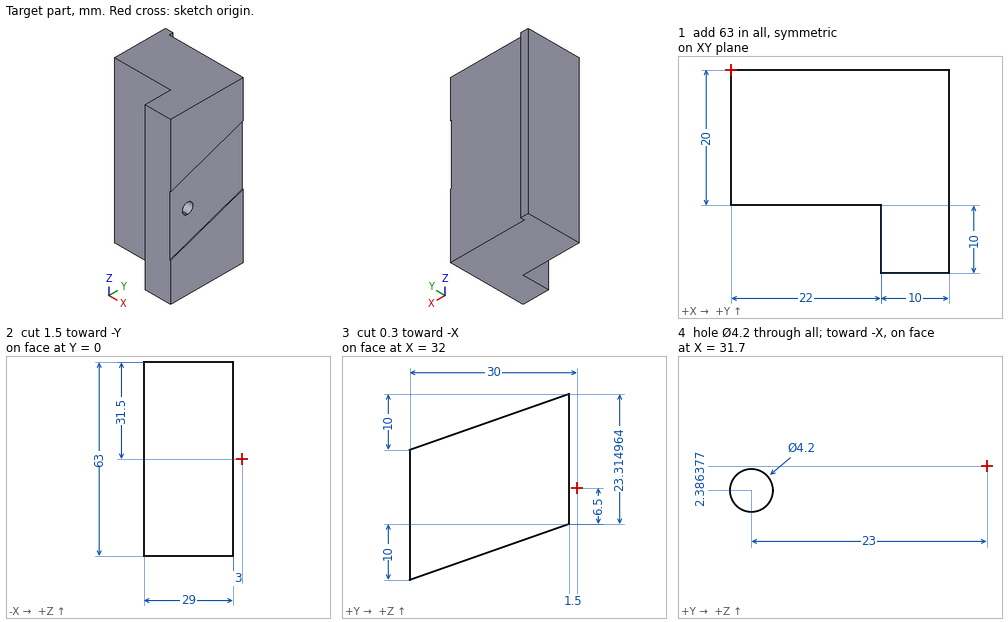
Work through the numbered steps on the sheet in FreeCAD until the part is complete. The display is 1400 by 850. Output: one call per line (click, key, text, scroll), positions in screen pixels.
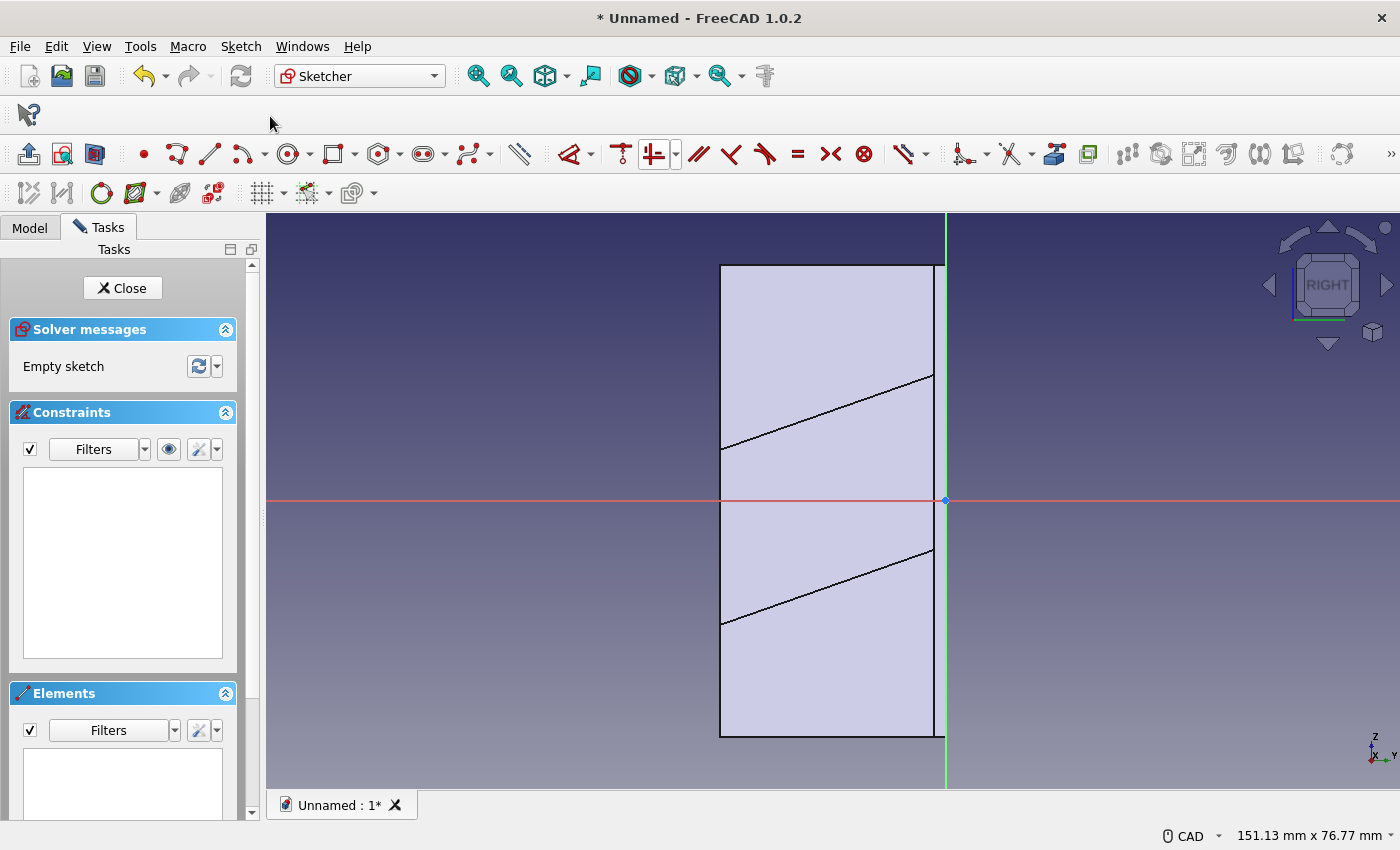
scroll(774, 521, up, 12)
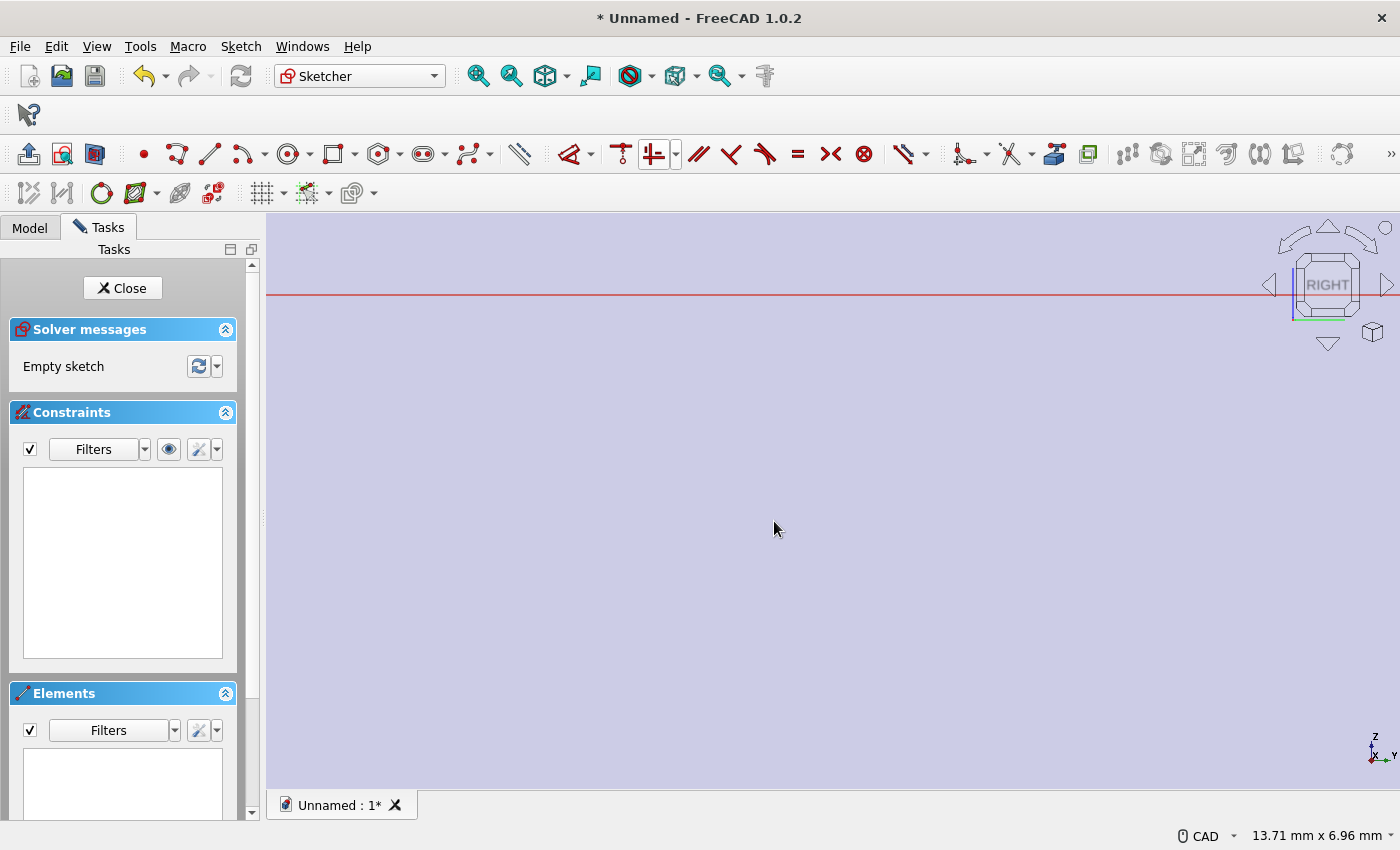
click(288, 154)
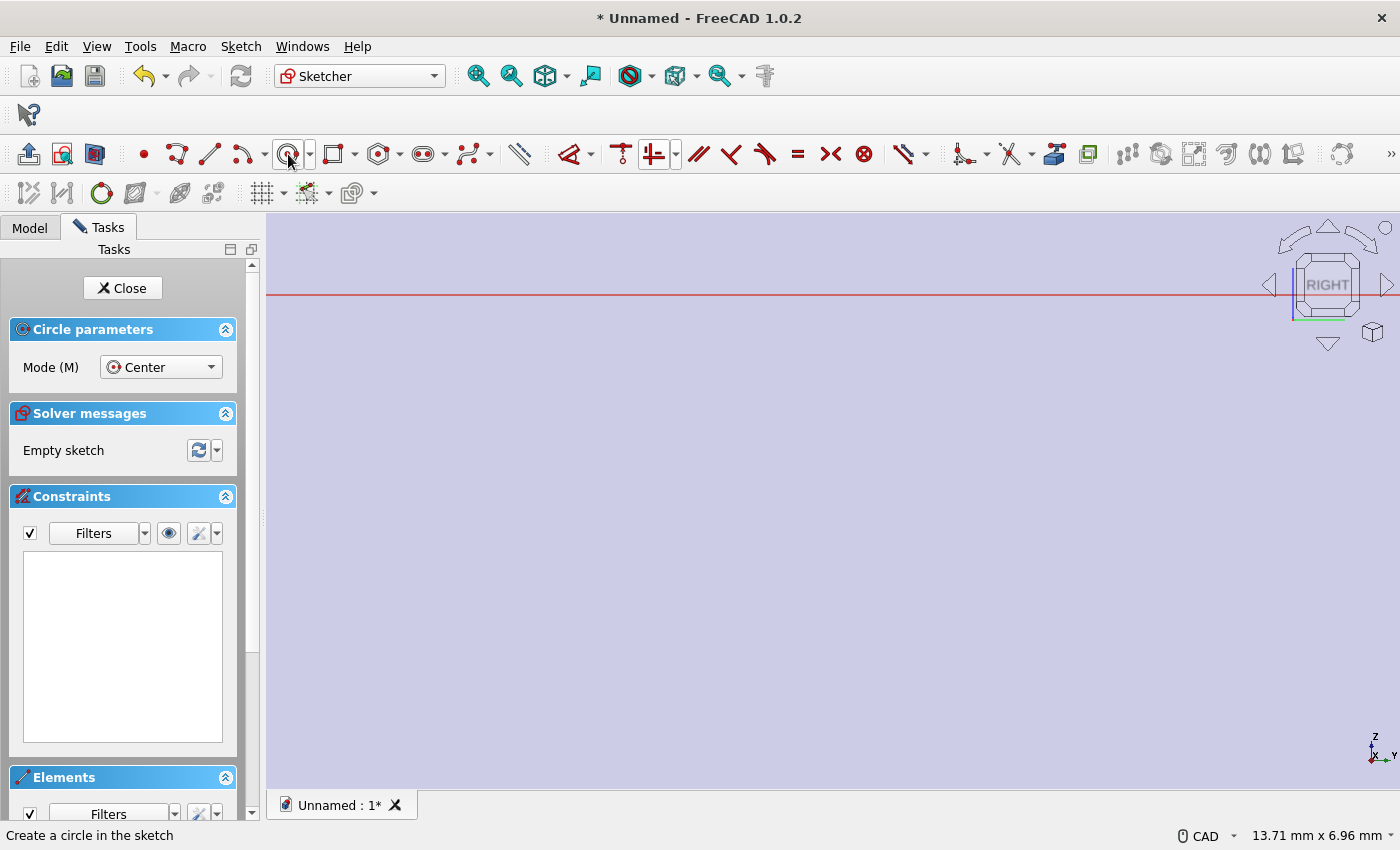
click(758, 493)
click(881, 370)
key(Escape)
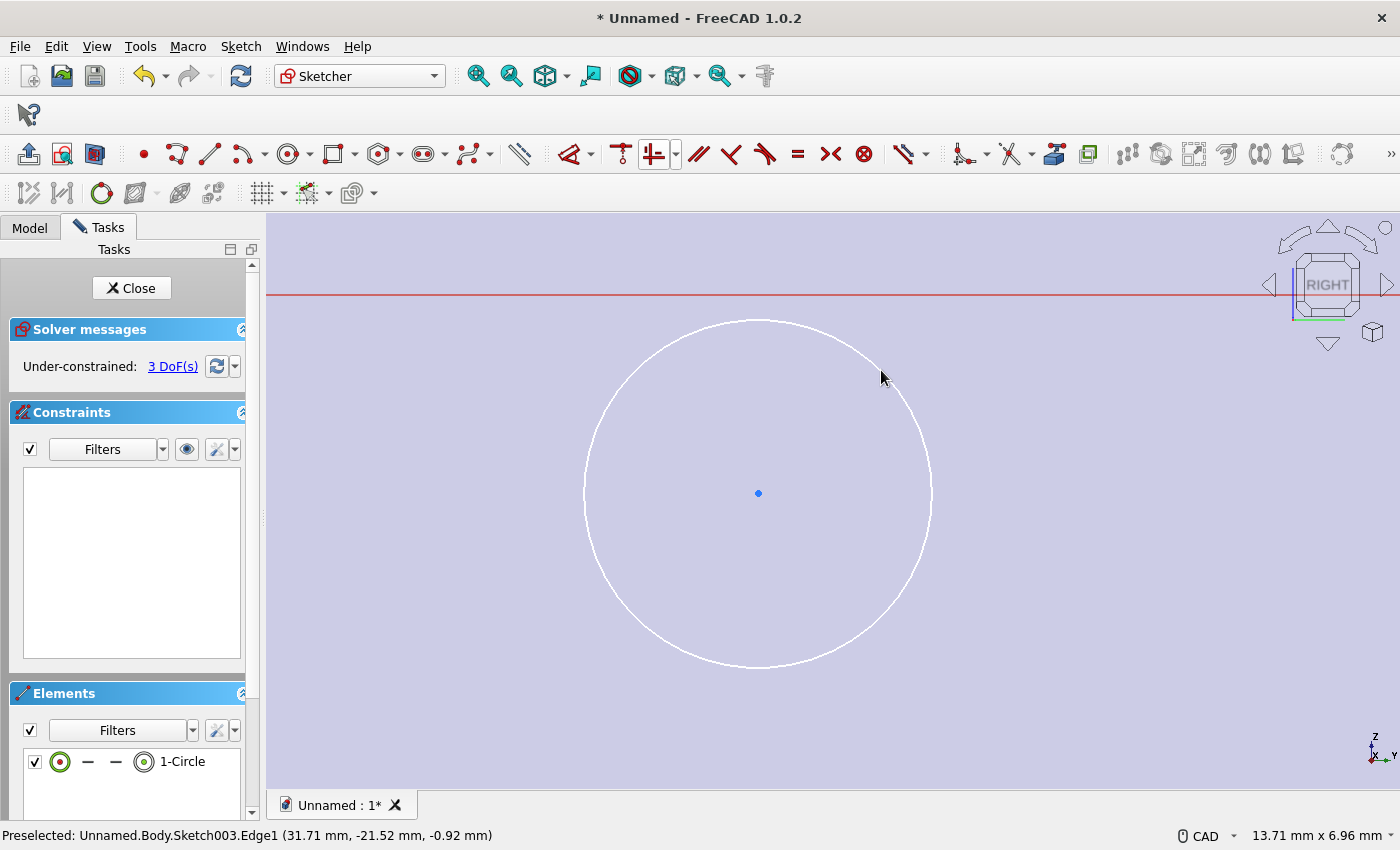
click(568, 154)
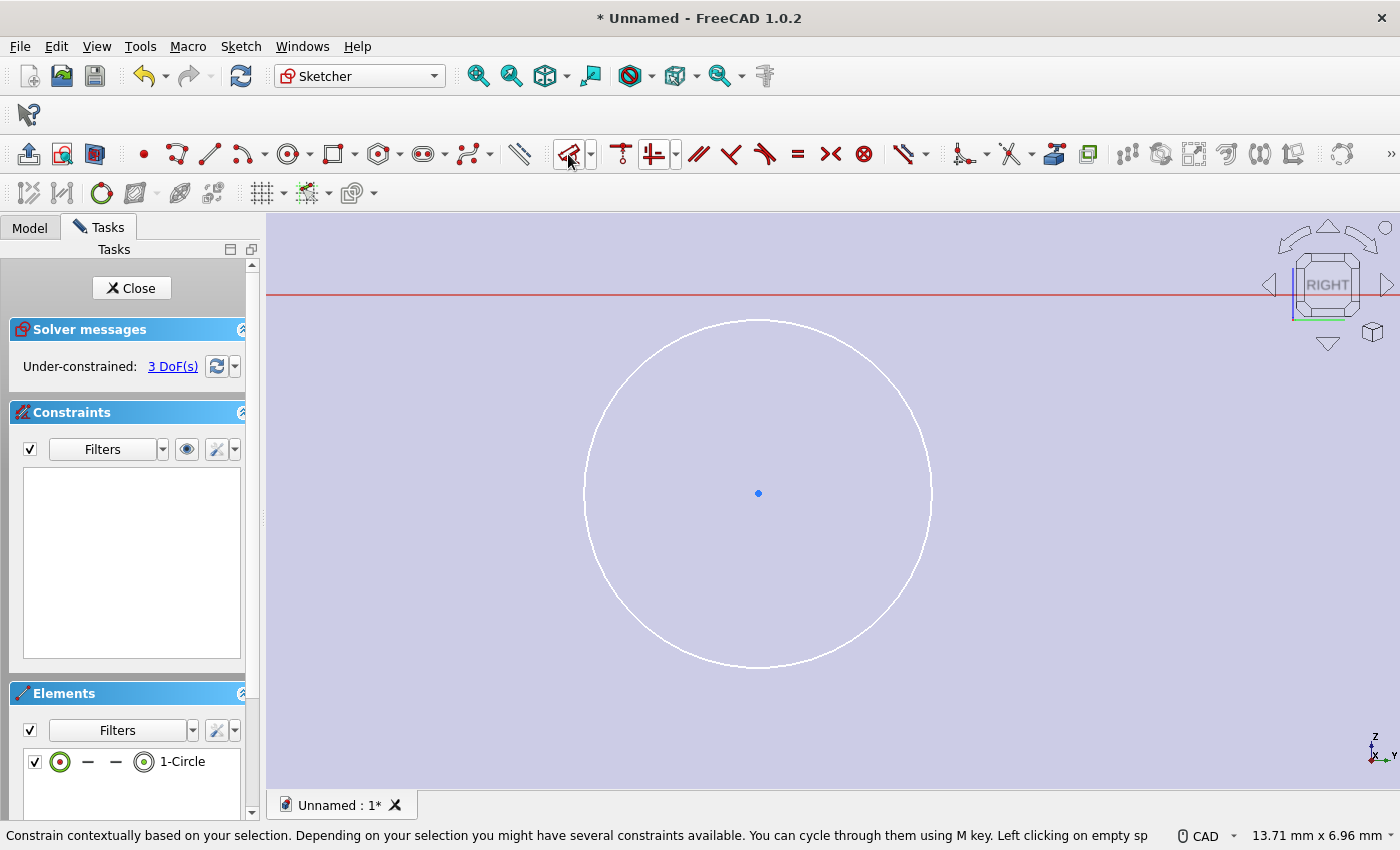
click(881, 371)
click(904, 348)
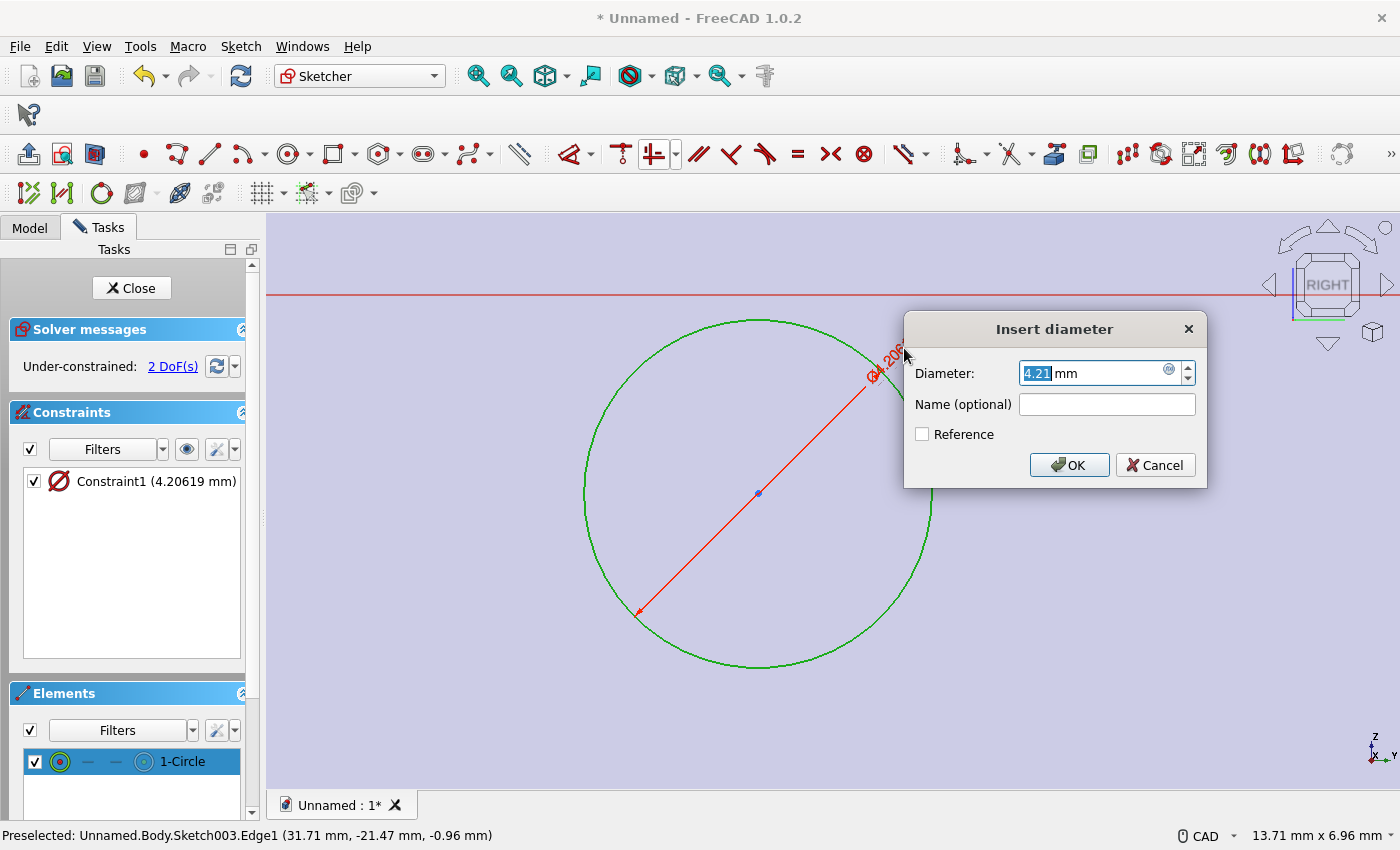
text(4.2)
key(Return)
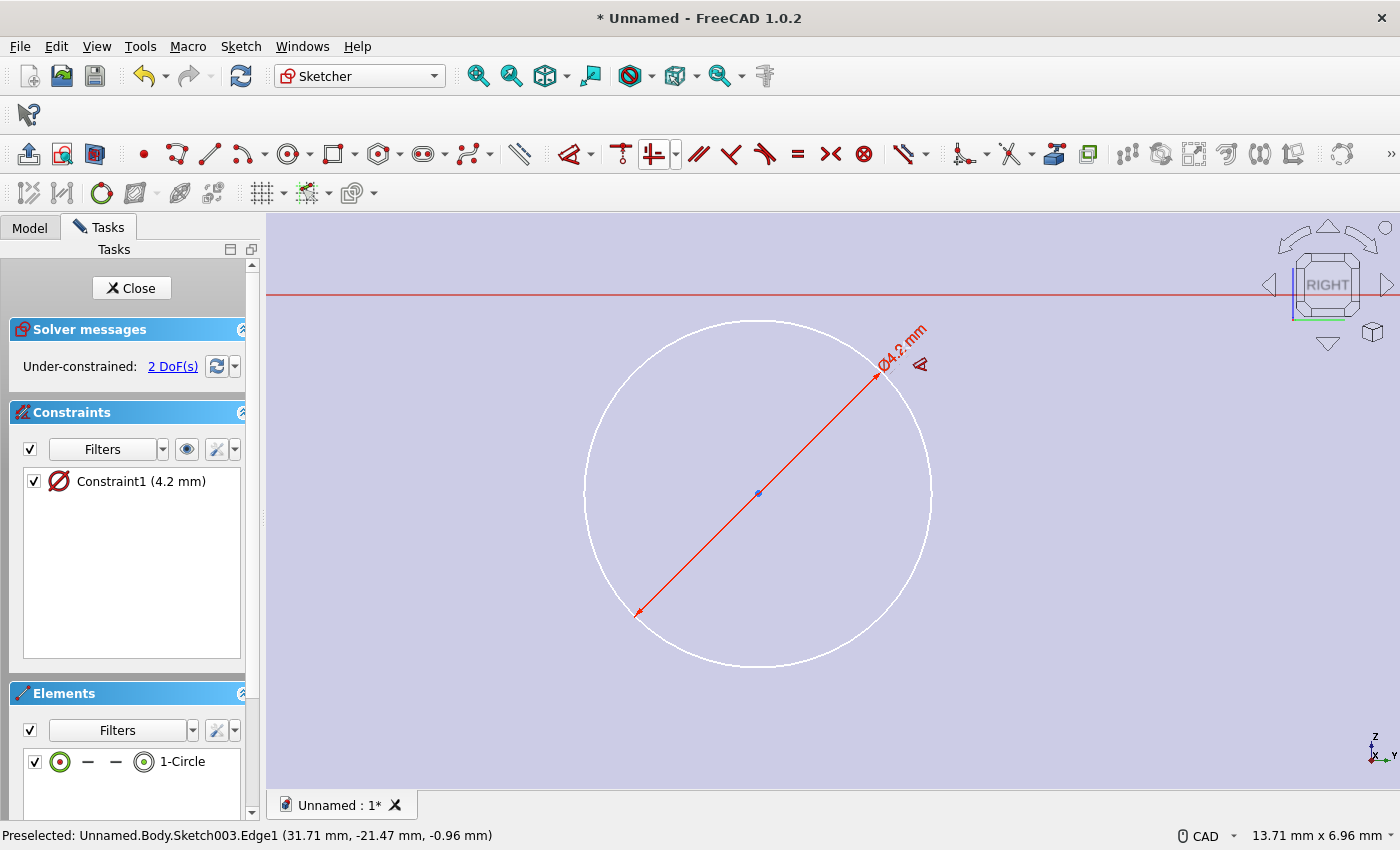
click(758, 494)
click(997, 261)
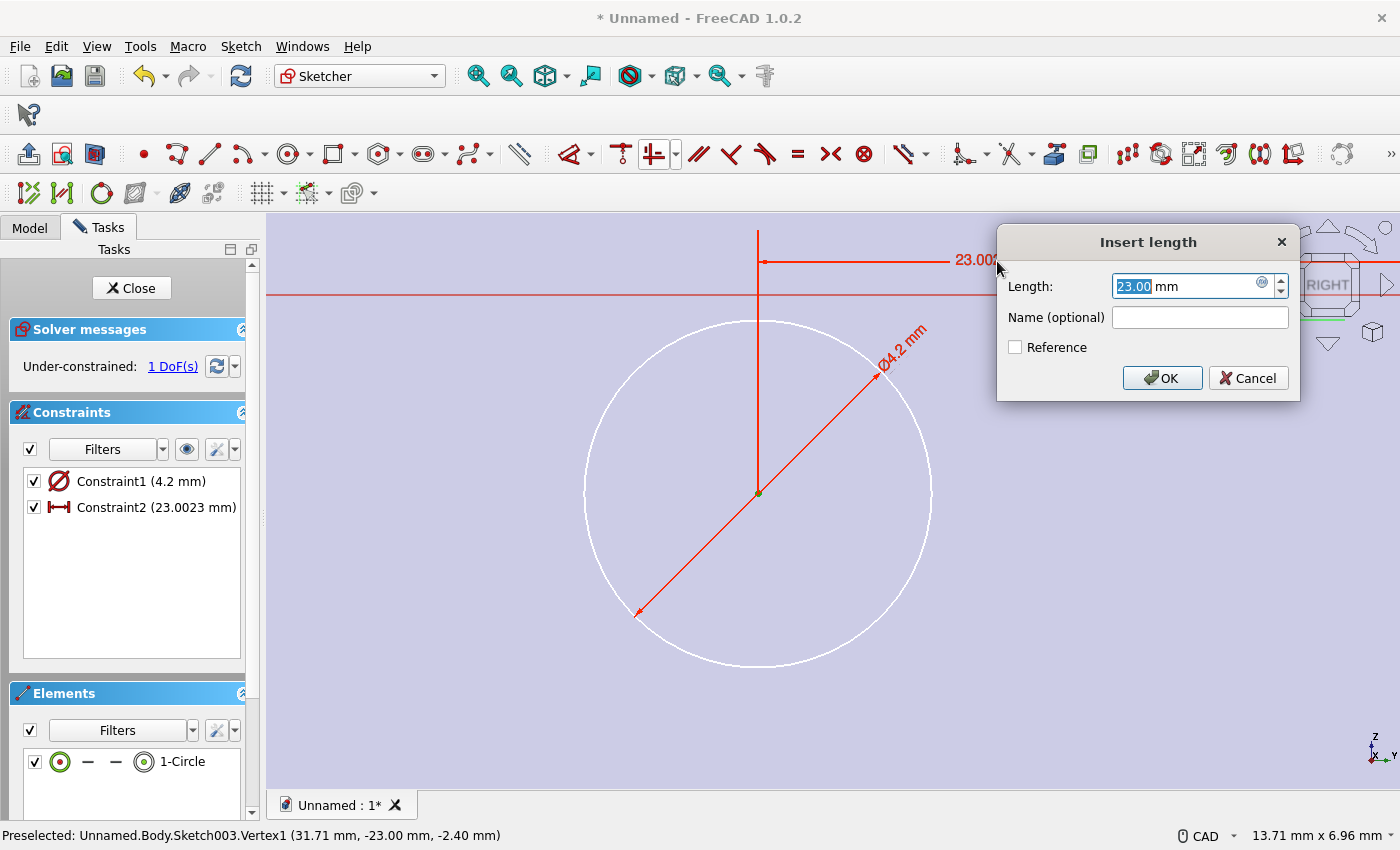
text(23)
key(Return)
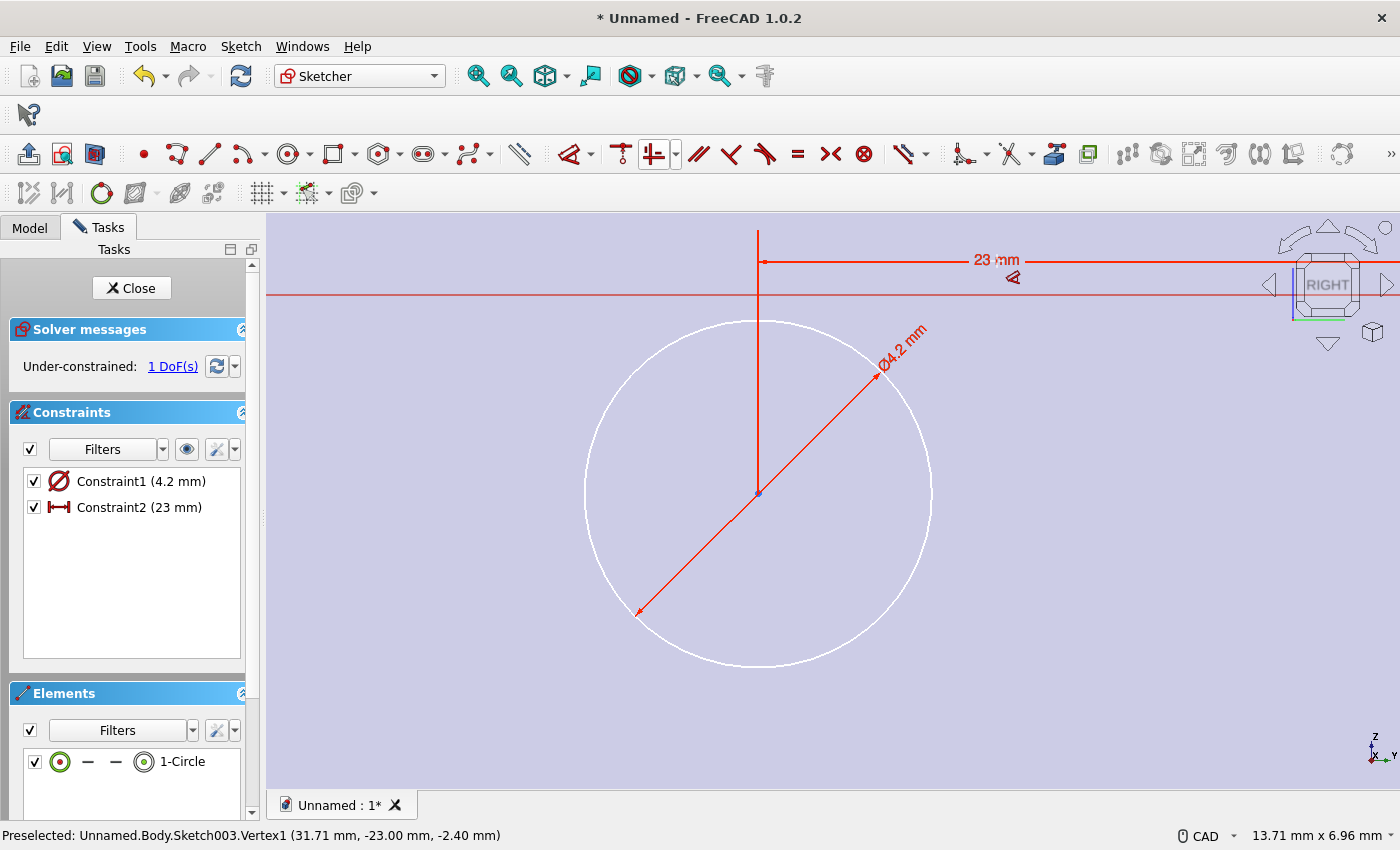
click(758, 494)
click(724, 395)